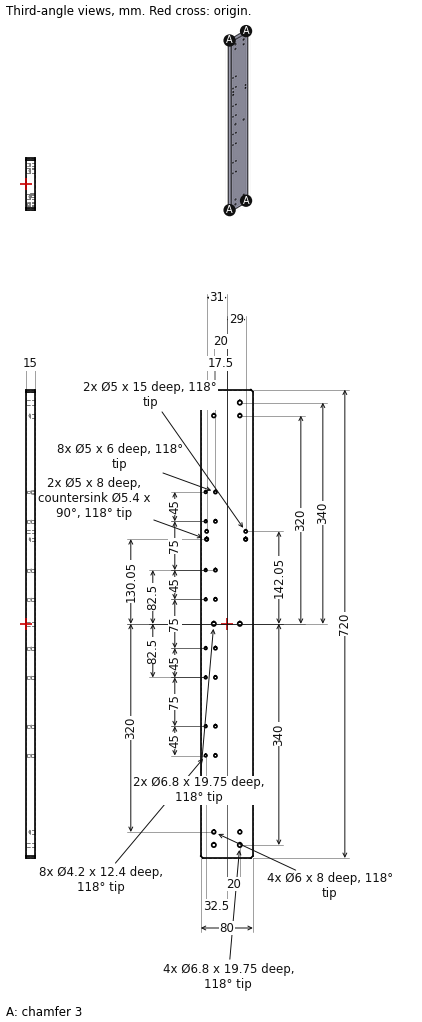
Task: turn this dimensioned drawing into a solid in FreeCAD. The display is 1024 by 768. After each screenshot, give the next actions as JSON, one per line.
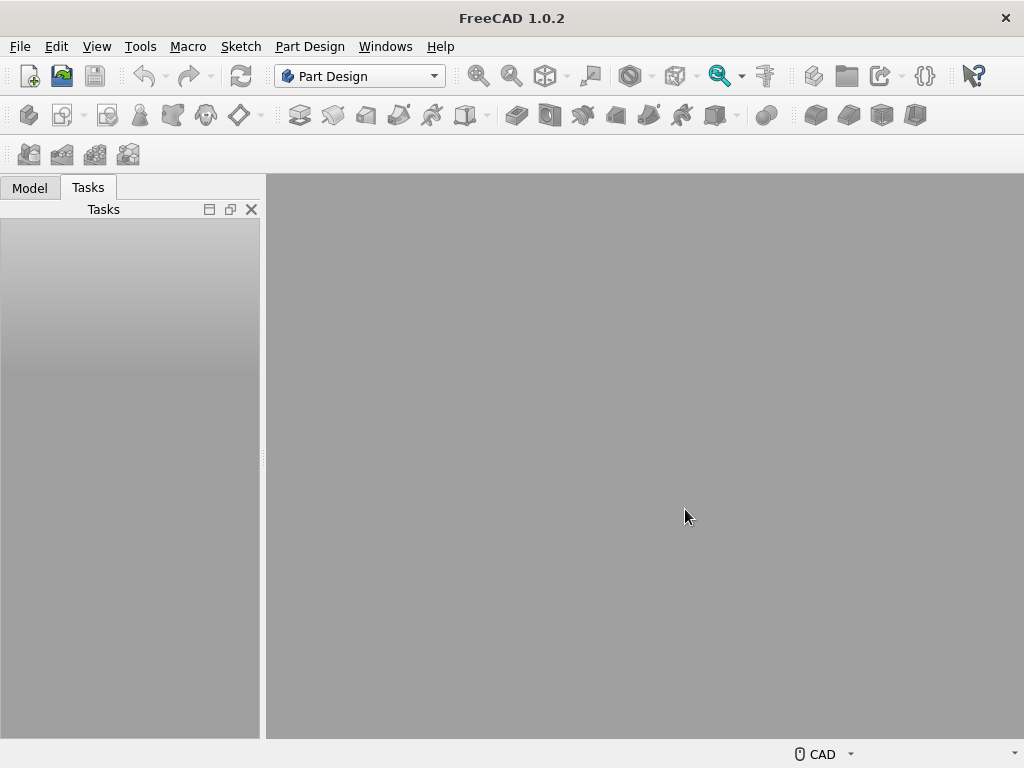
{"action": "key", "text": "ctrl+n"}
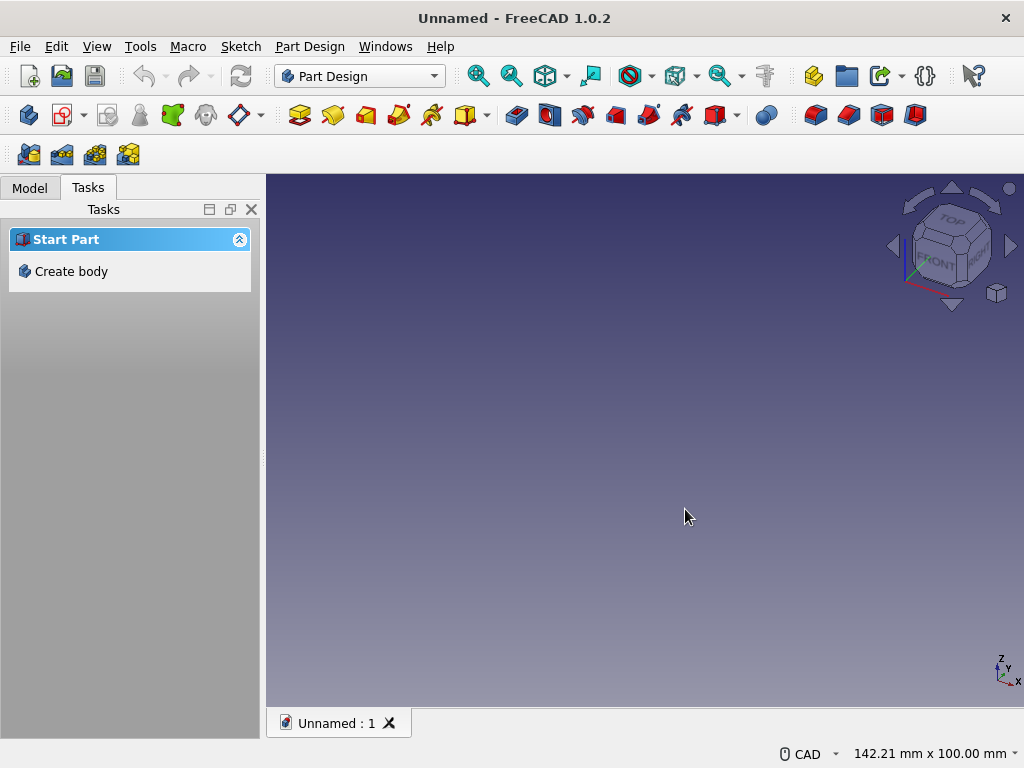
{"action": "left_click", "coordinate": [62, 116]}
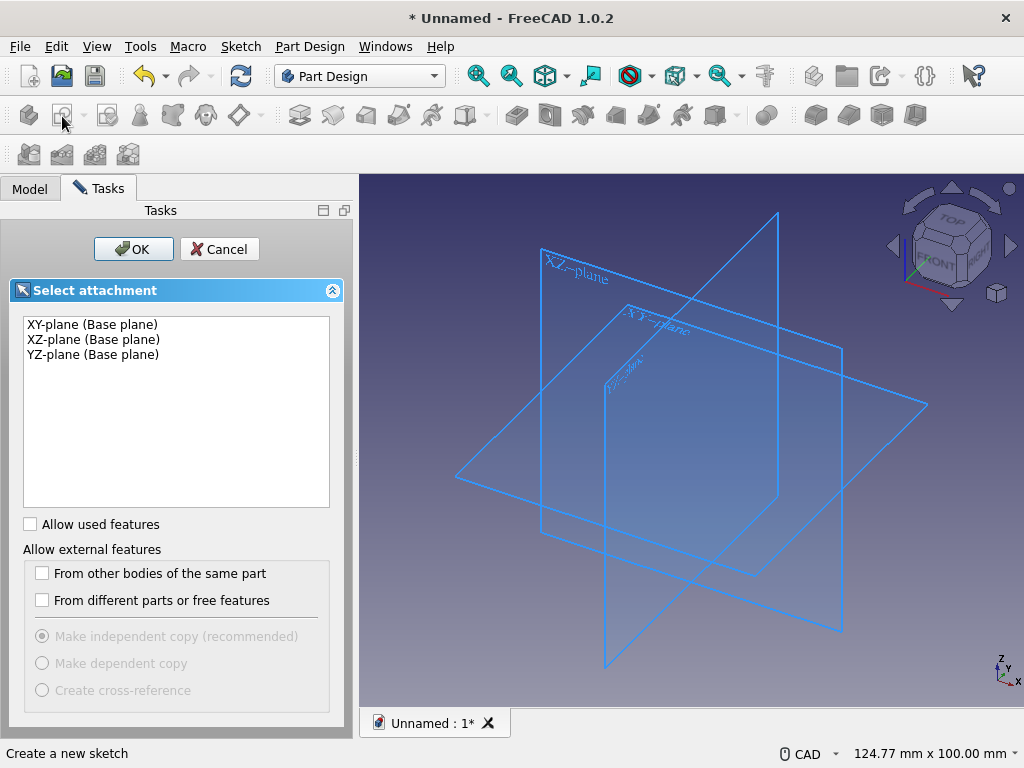
{"action": "left_click", "coordinate": [84, 354]}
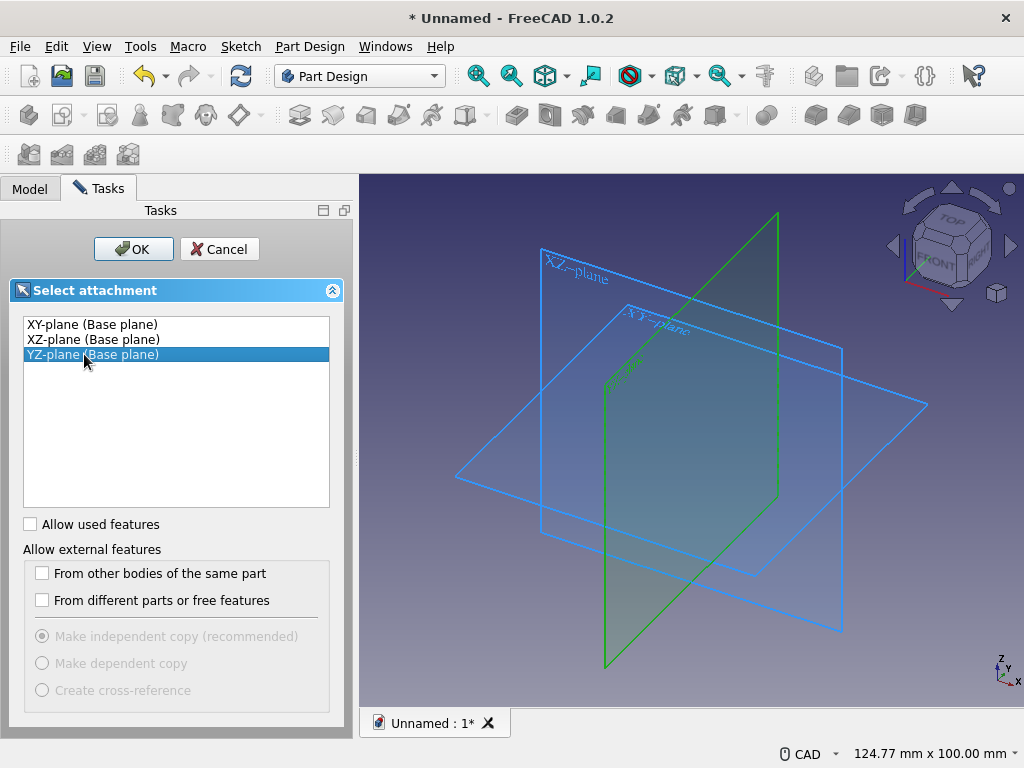
{"action": "left_click", "coordinate": [134, 249]}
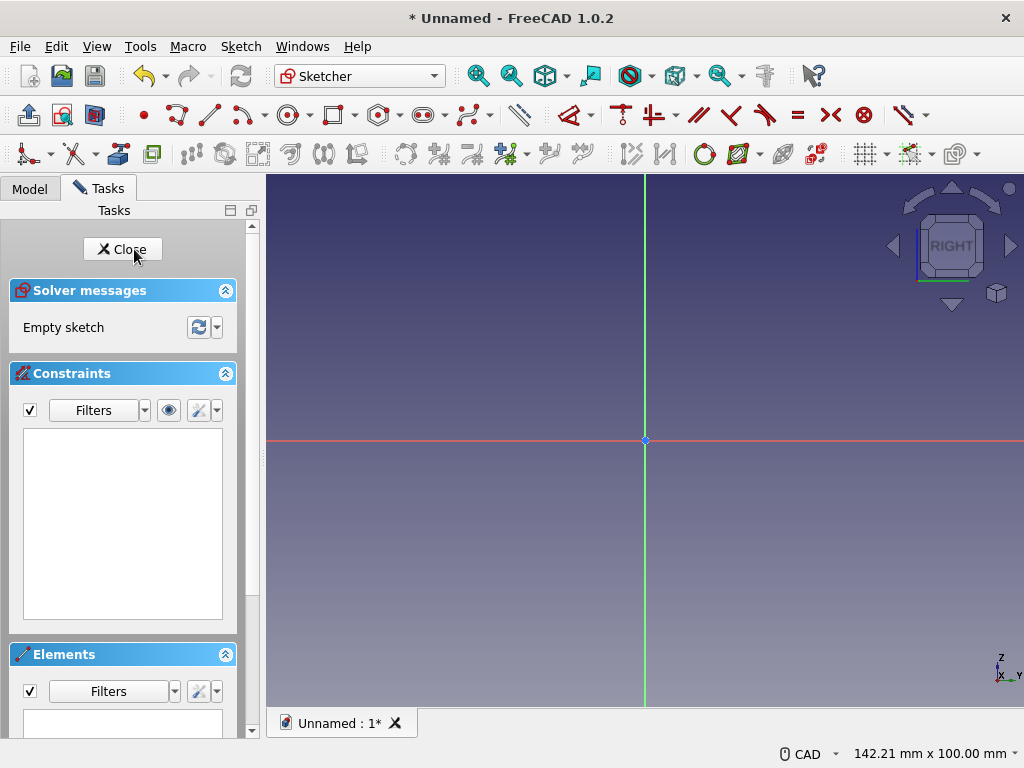
{"action": "scroll", "coordinate": [570, 440], "scroll_direction": "down", "scroll_amount": 12}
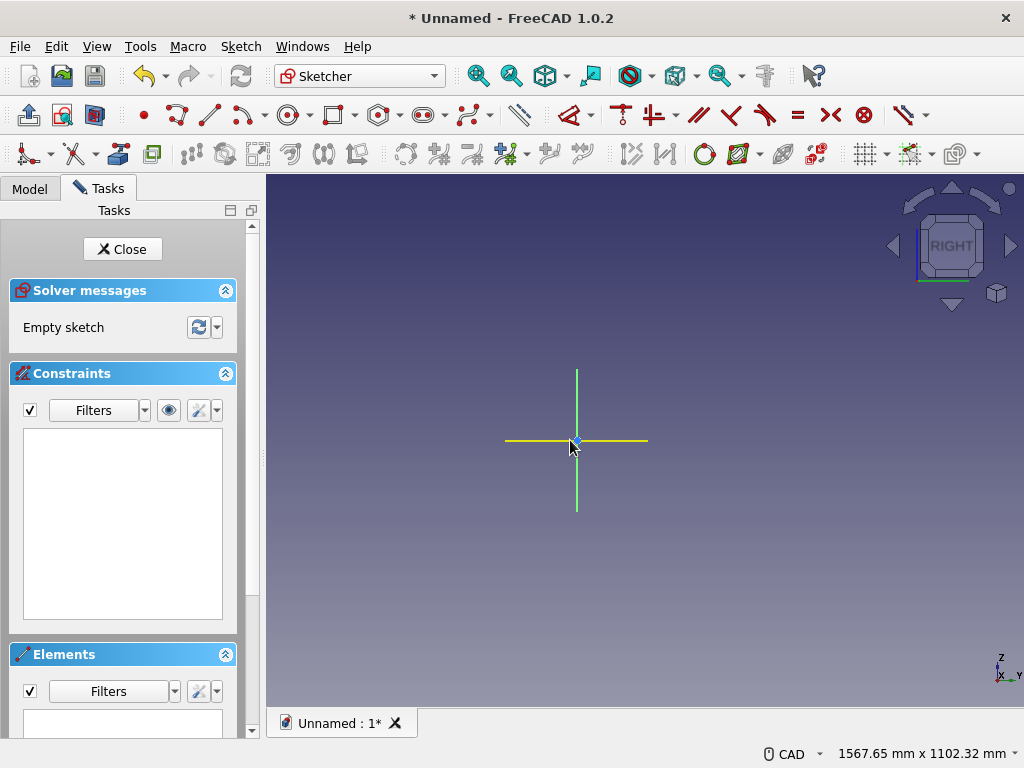
{"action": "key", "text": "g v"}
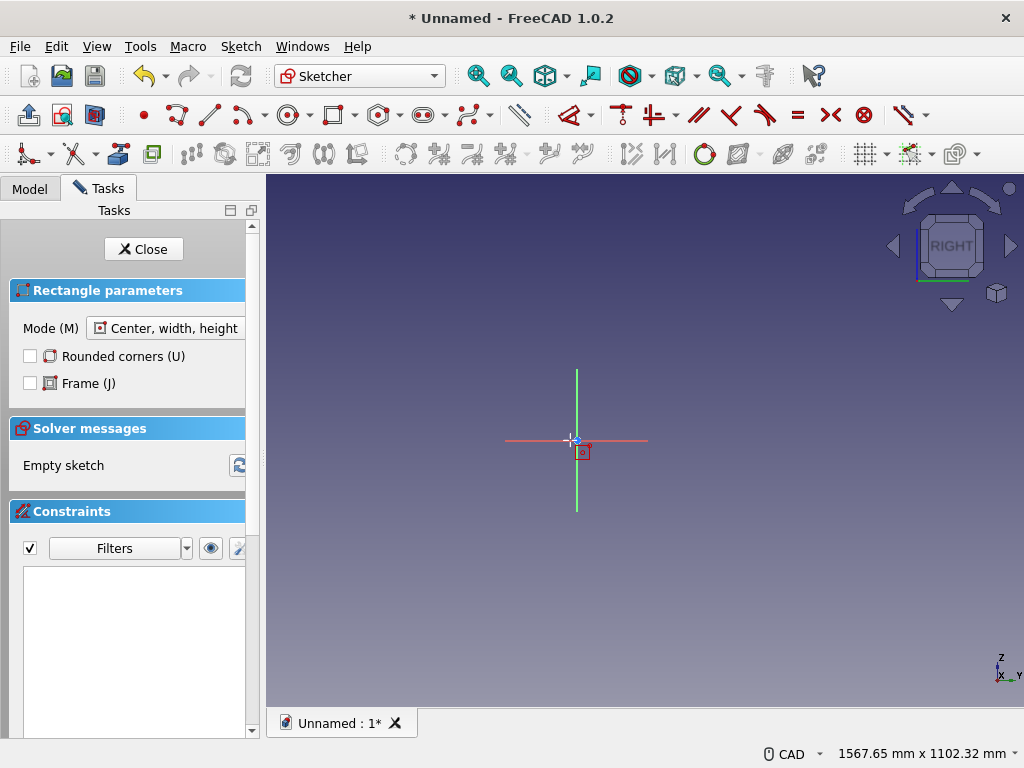
{"action": "left_click", "coordinate": [577, 440]}
{"action": "mouse_move", "coordinate": [597, 266]}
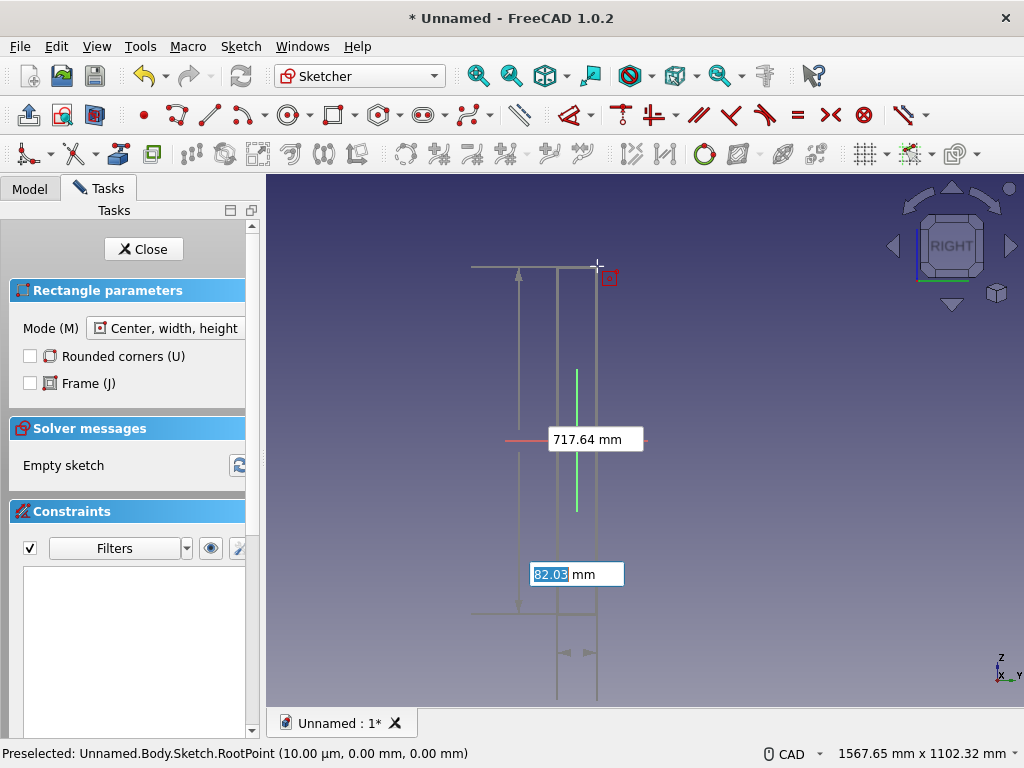
{"action": "type", "text": "80"}
{"action": "key", "text": "Tab"}
{"action": "type", "text": "720"}
{"action": "key", "text": "Return"}
{"action": "key", "text": "Escape"}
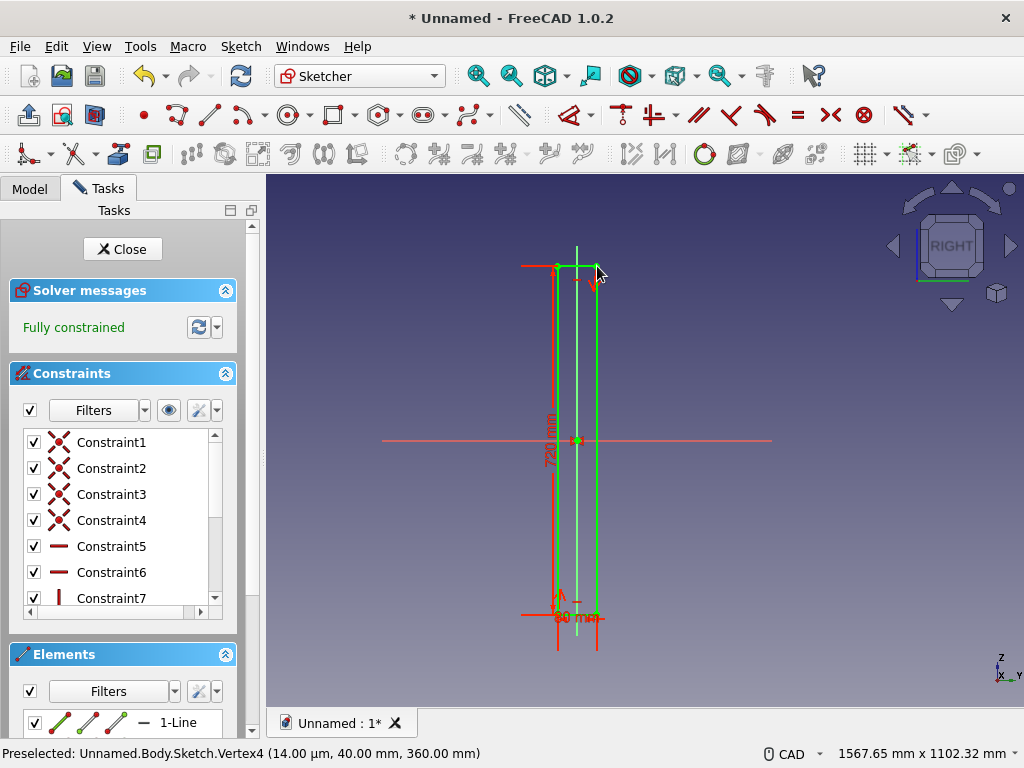
{"action": "left_click", "coordinate": [123, 249]}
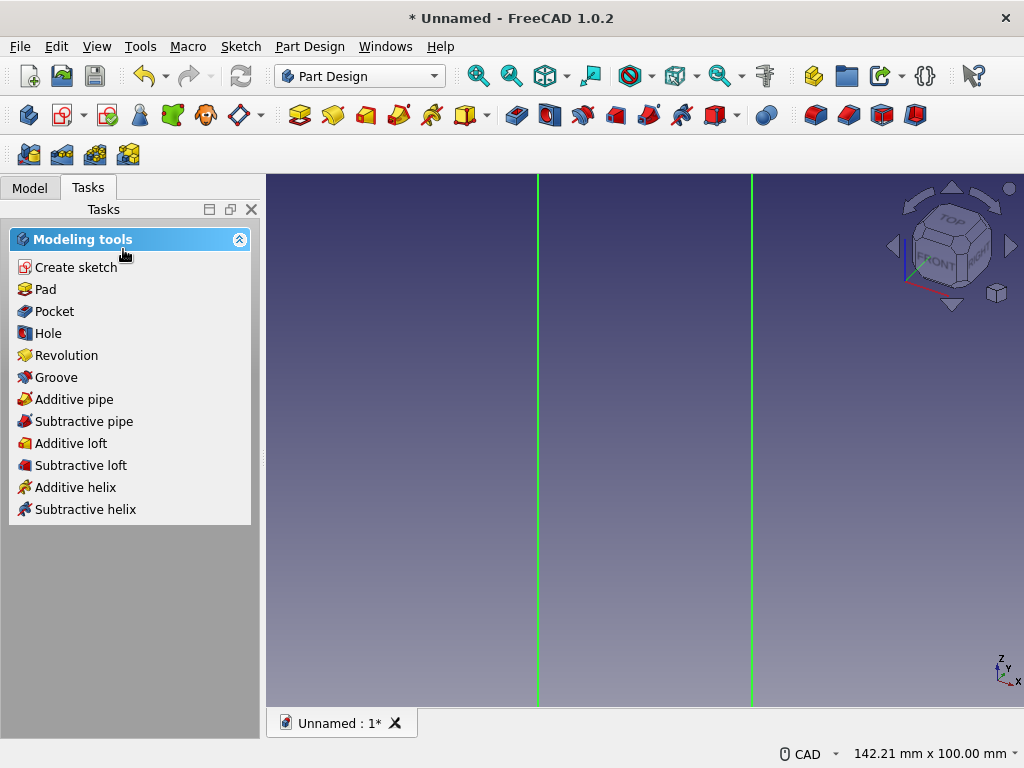
{"action": "left_click", "coordinate": [300, 116]}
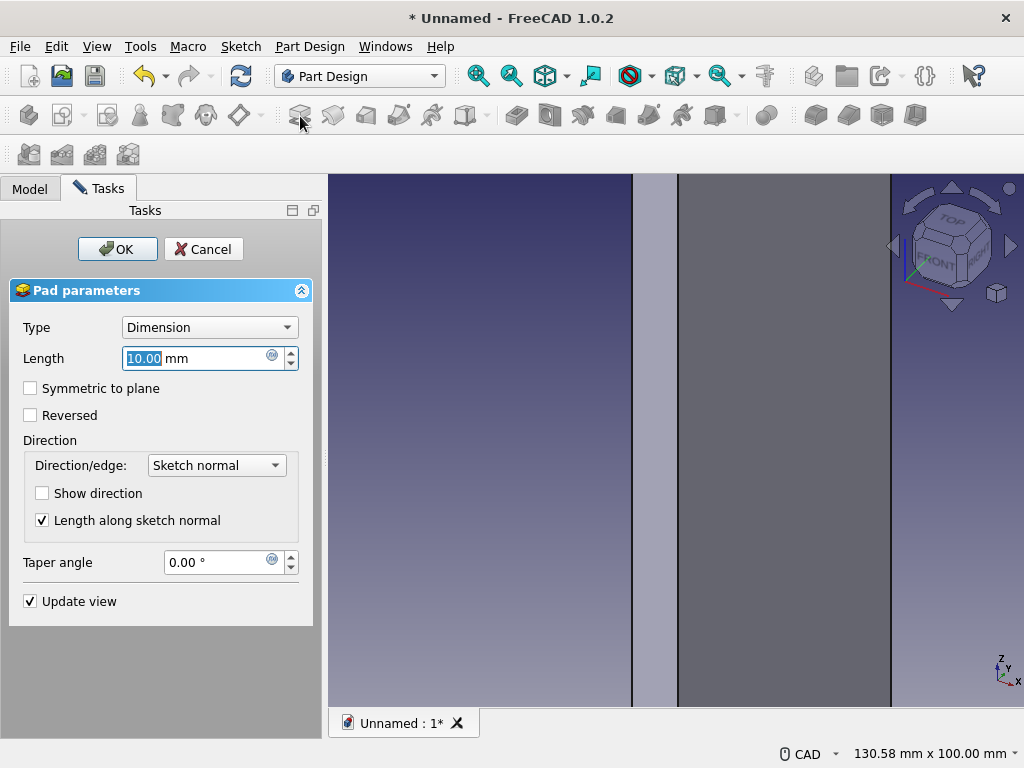
{"action": "type", "text": "15"}
{"action": "key", "text": "Tab"}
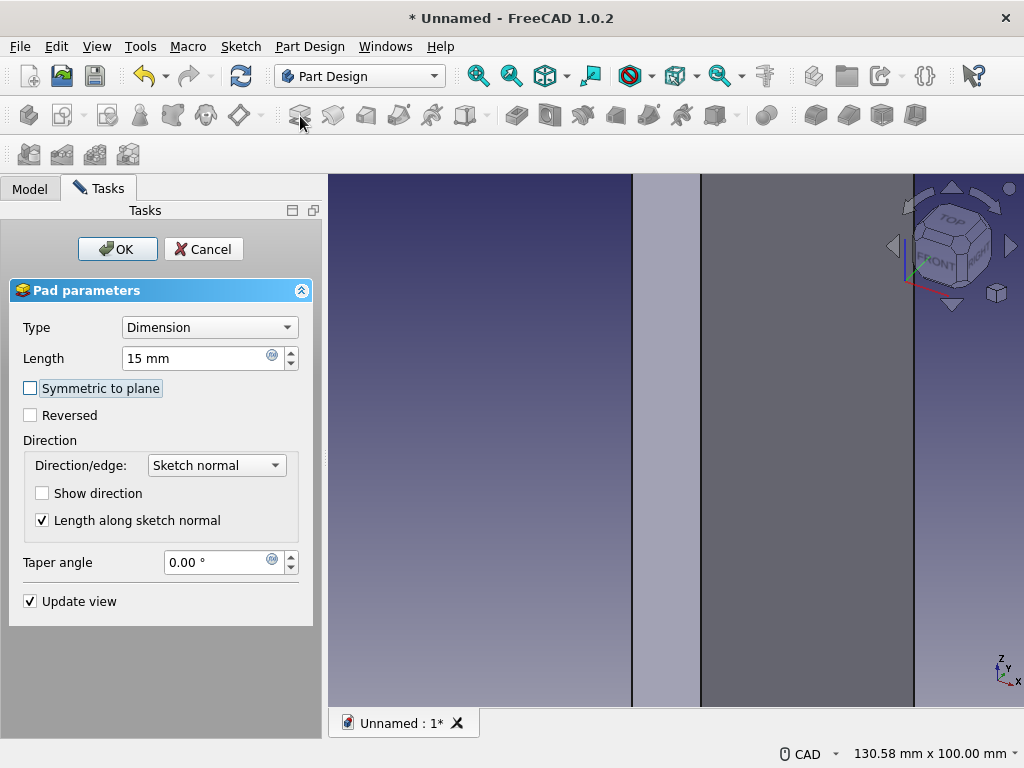
{"action": "left_click", "coordinate": [118, 249]}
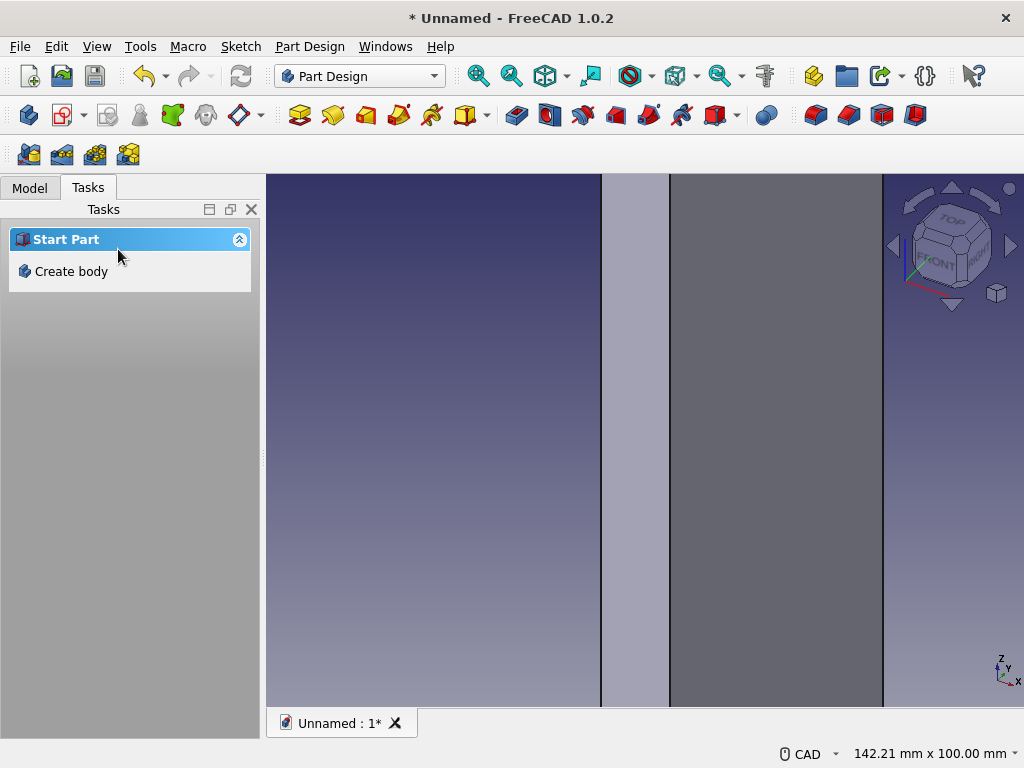
{"action": "key", "text": "v f"}